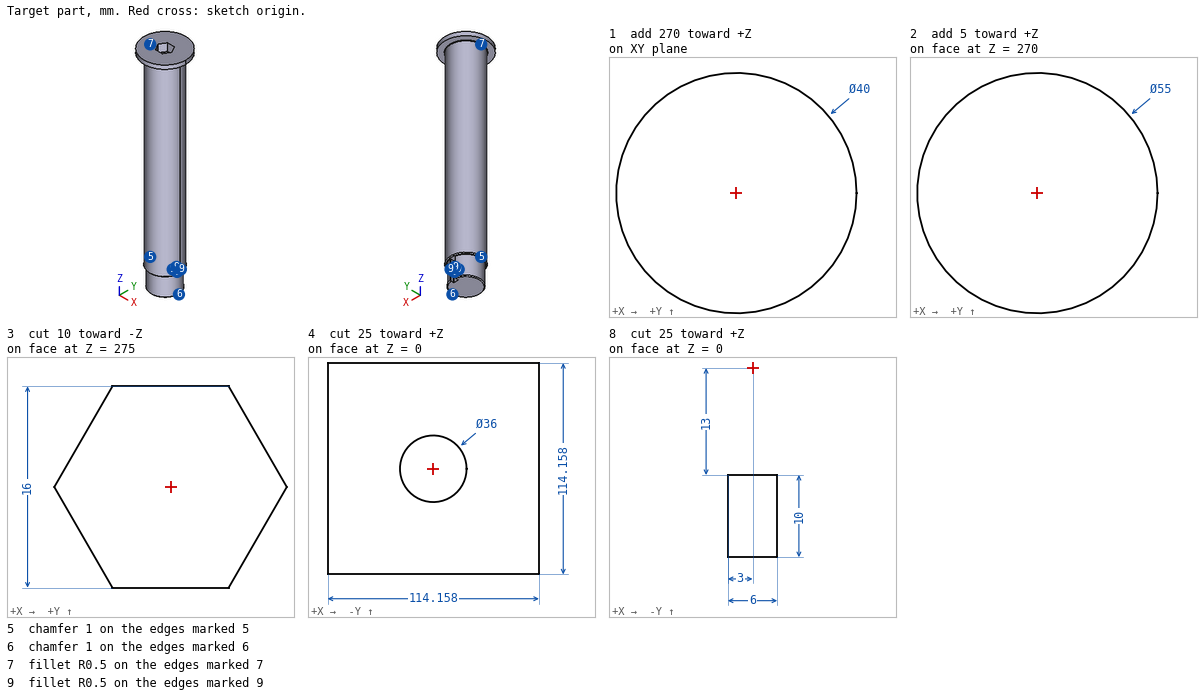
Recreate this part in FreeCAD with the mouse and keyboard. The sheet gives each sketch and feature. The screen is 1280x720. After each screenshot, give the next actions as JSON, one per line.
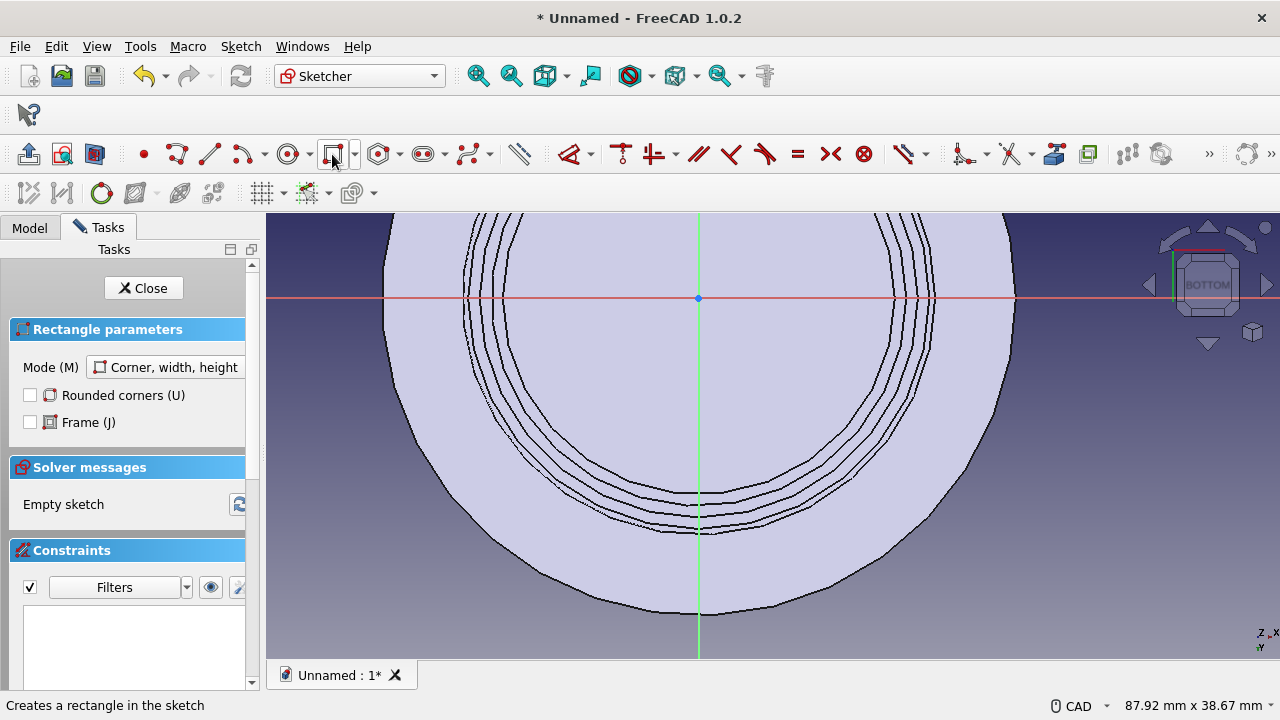
{"action": "left_click", "coordinate": [664, 448]}
{"action": "mouse_move", "coordinate": [733, 564]}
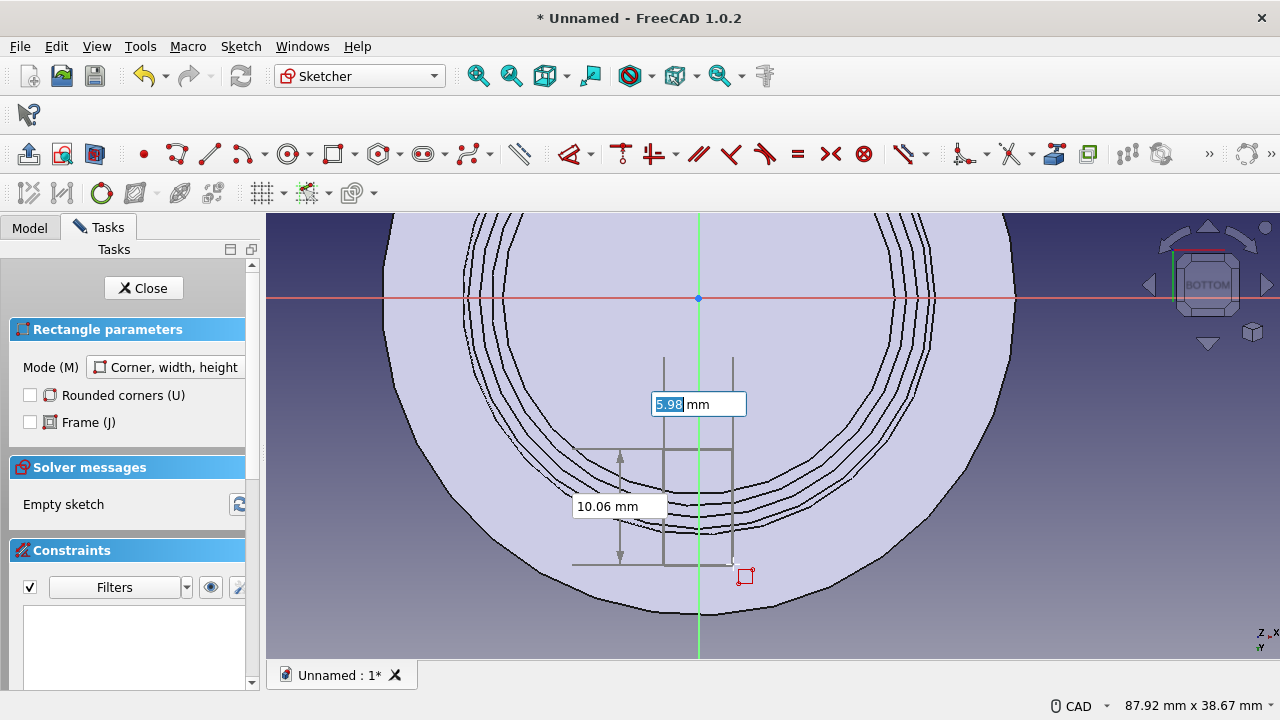
{"action": "type", "text": "6"}
{"action": "key", "text": "Tab"}
{"action": "type", "text": "10"}
{"action": "key", "text": "Return"}
{"action": "key", "text": "Escape"}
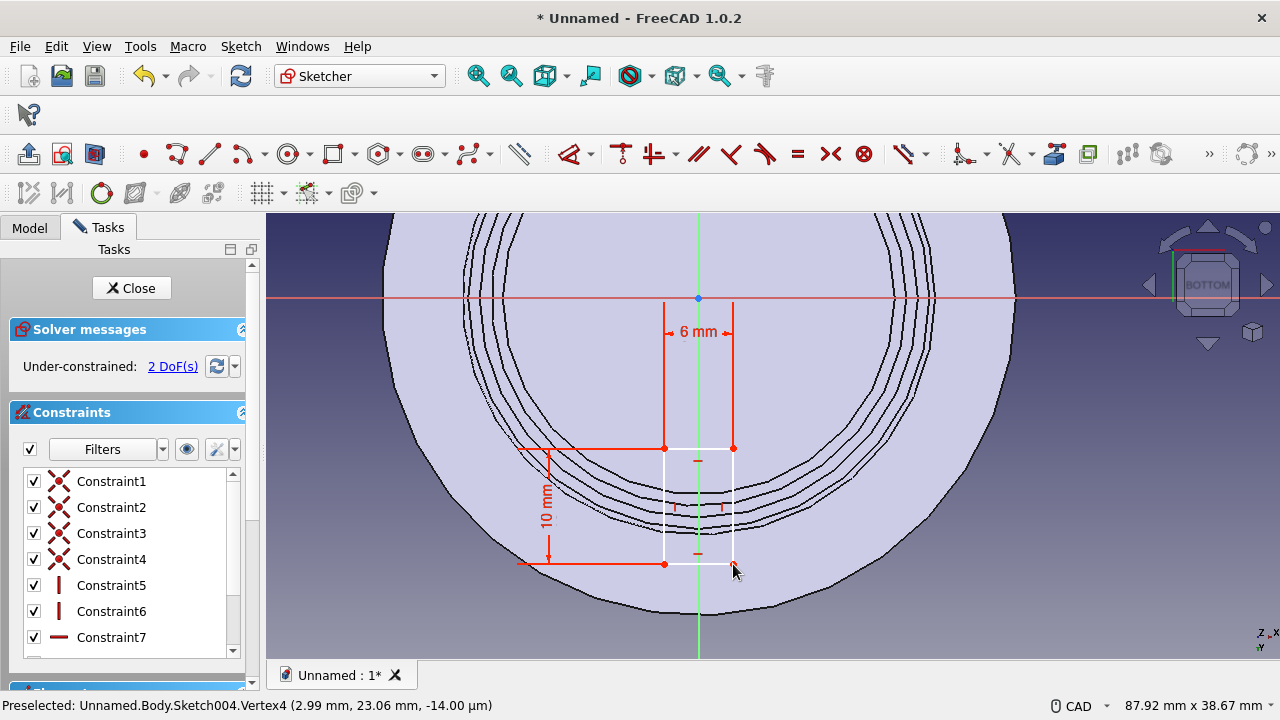
{"action": "left_click", "coordinate": [568, 154]}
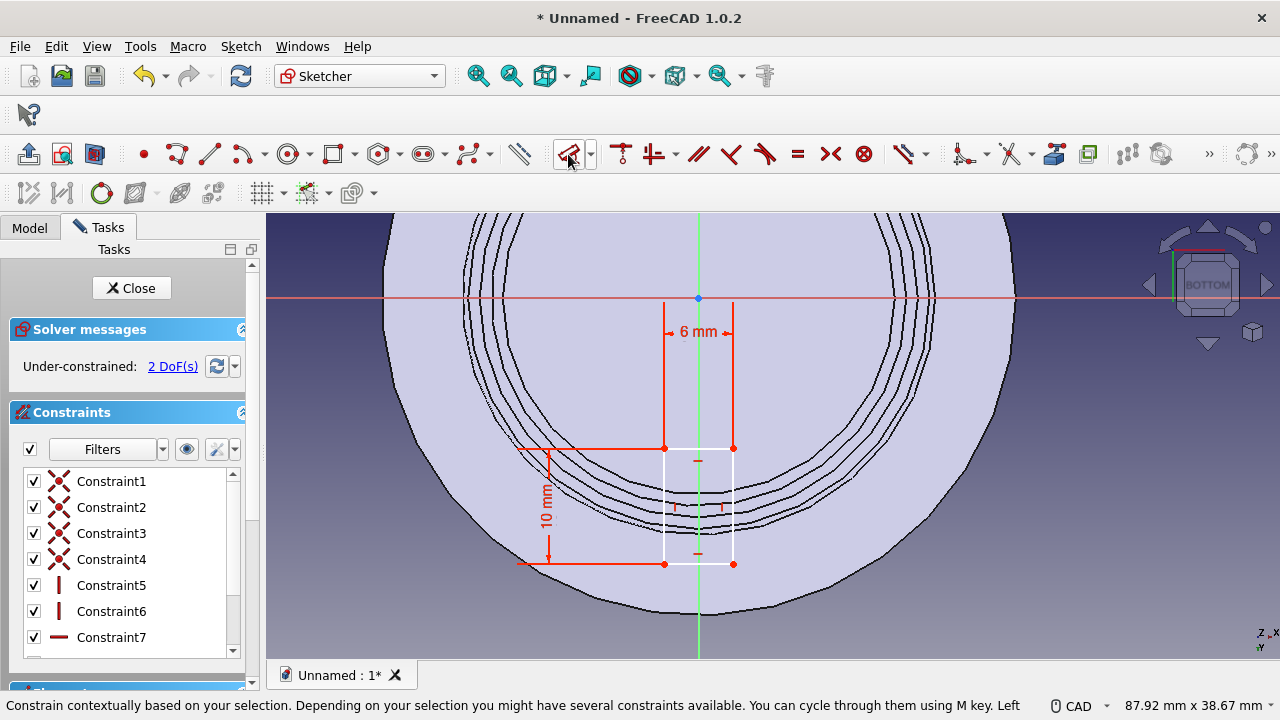
{"action": "left_click", "coordinate": [664, 449]}
{"action": "left_click", "coordinate": [681, 264]}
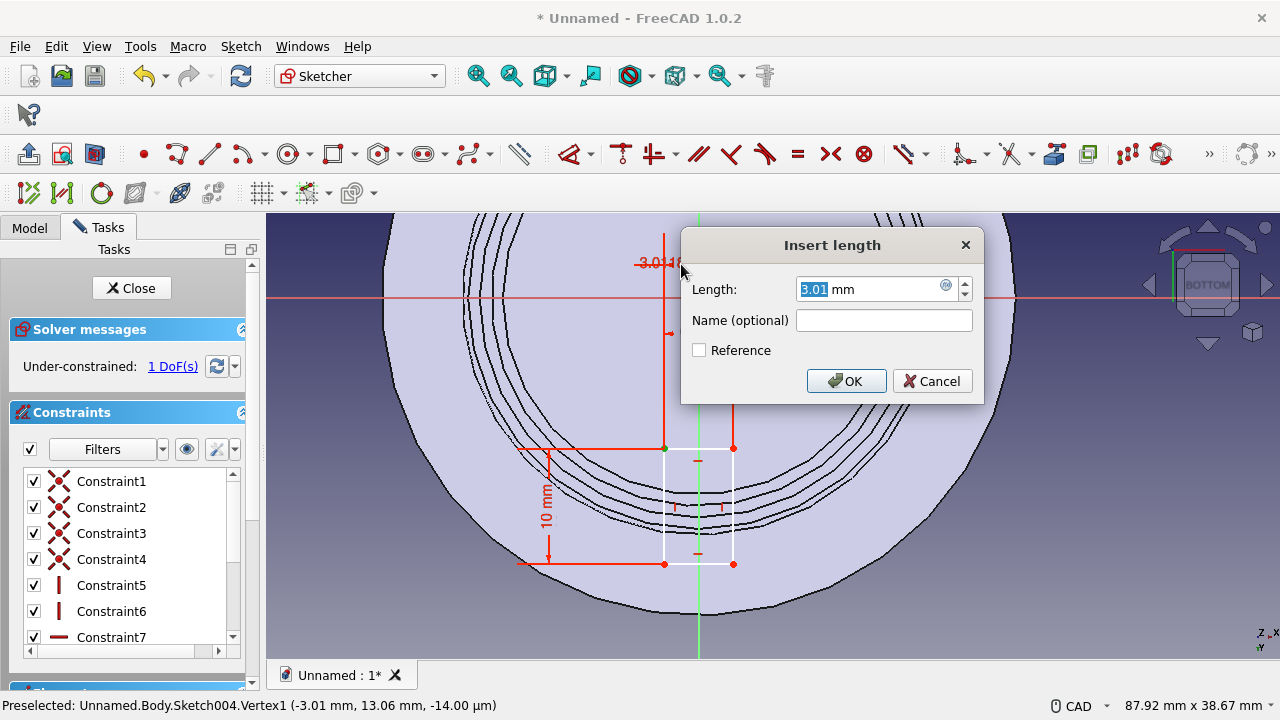
{"action": "type", "text": "3"}
{"action": "key", "text": "Return"}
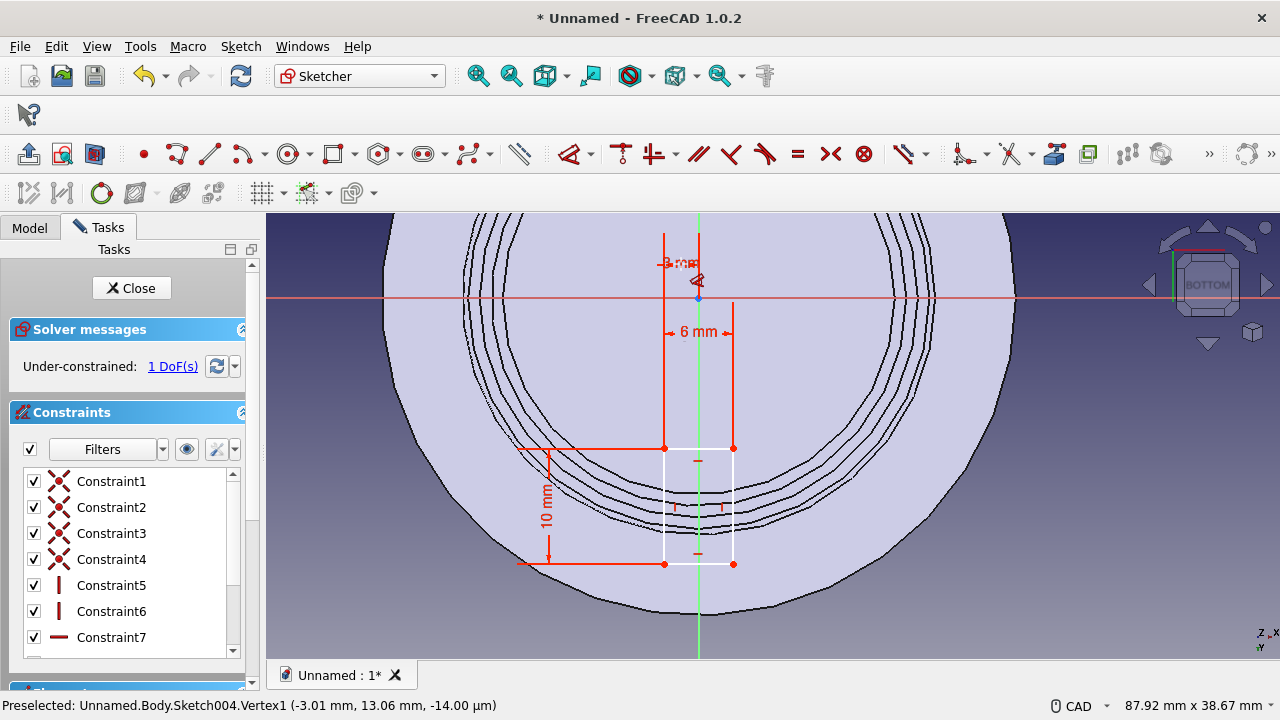
{"action": "left_click", "coordinate": [664, 449]}
{"action": "left_click", "coordinate": [630, 374]}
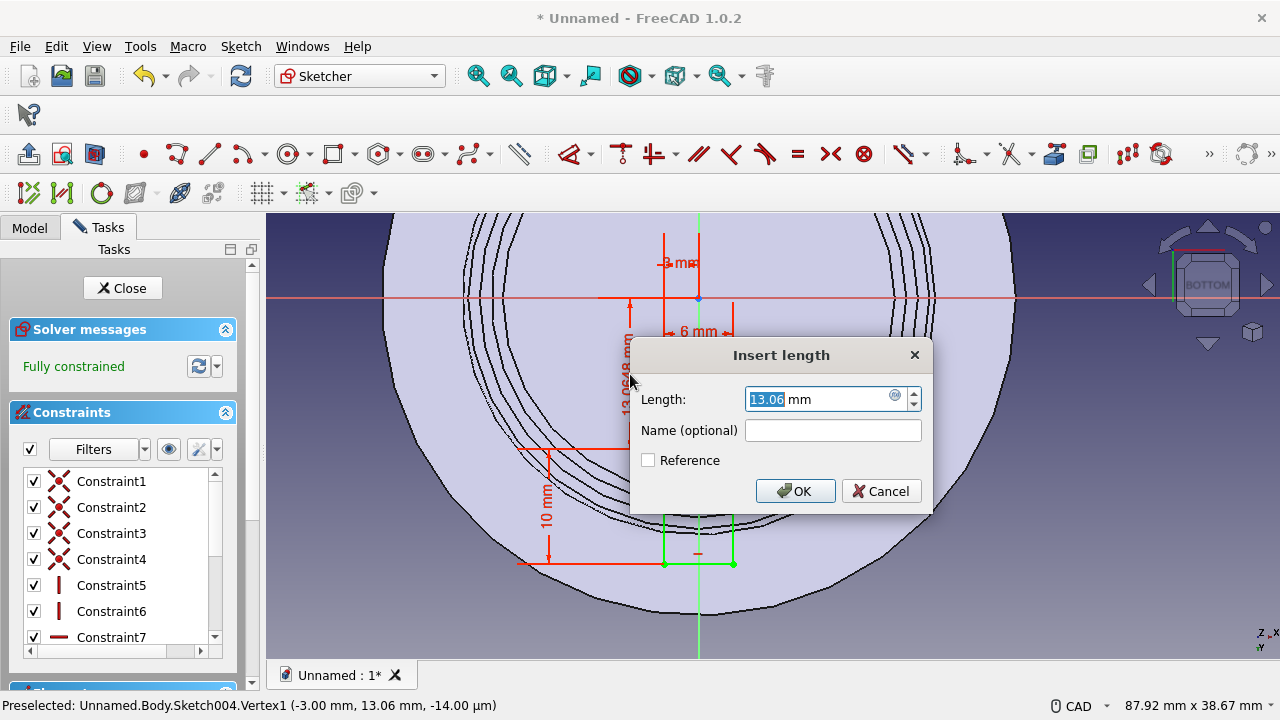
{"action": "type", "text": "13"}
{"action": "key", "text": "Return"}
{"action": "key", "text": "Escape"}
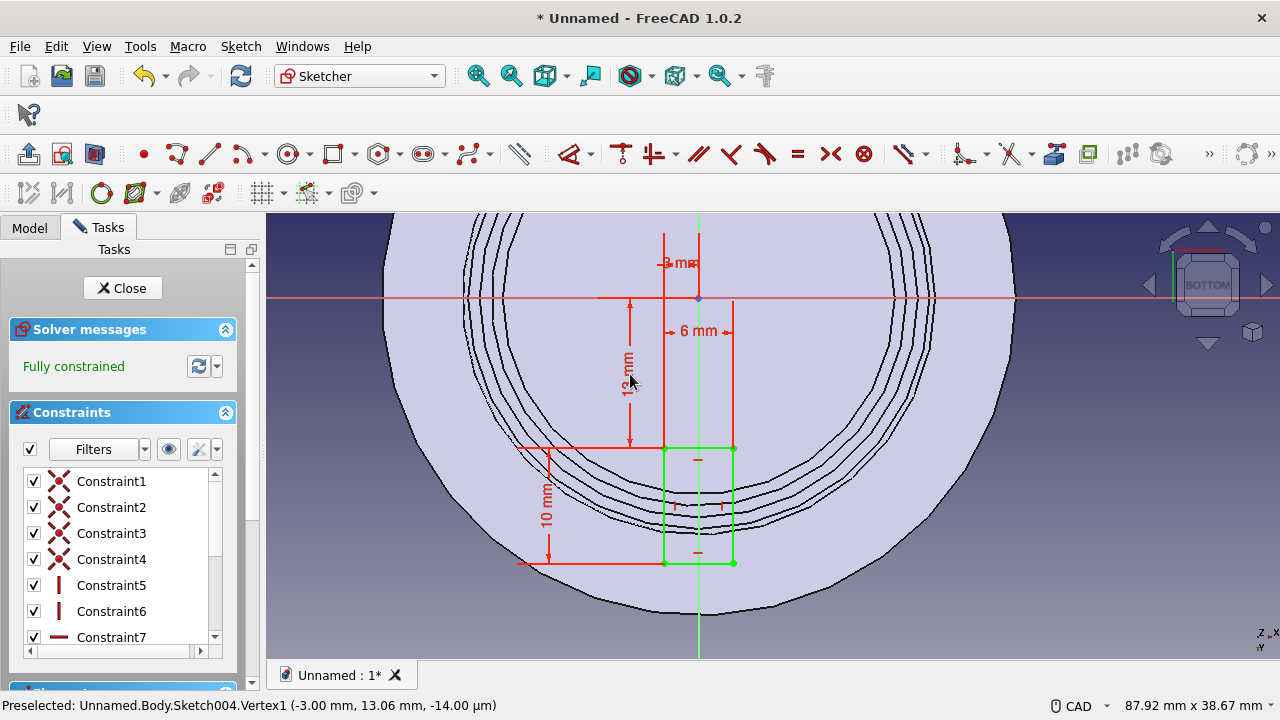
{"action": "left_click", "coordinate": [123, 288]}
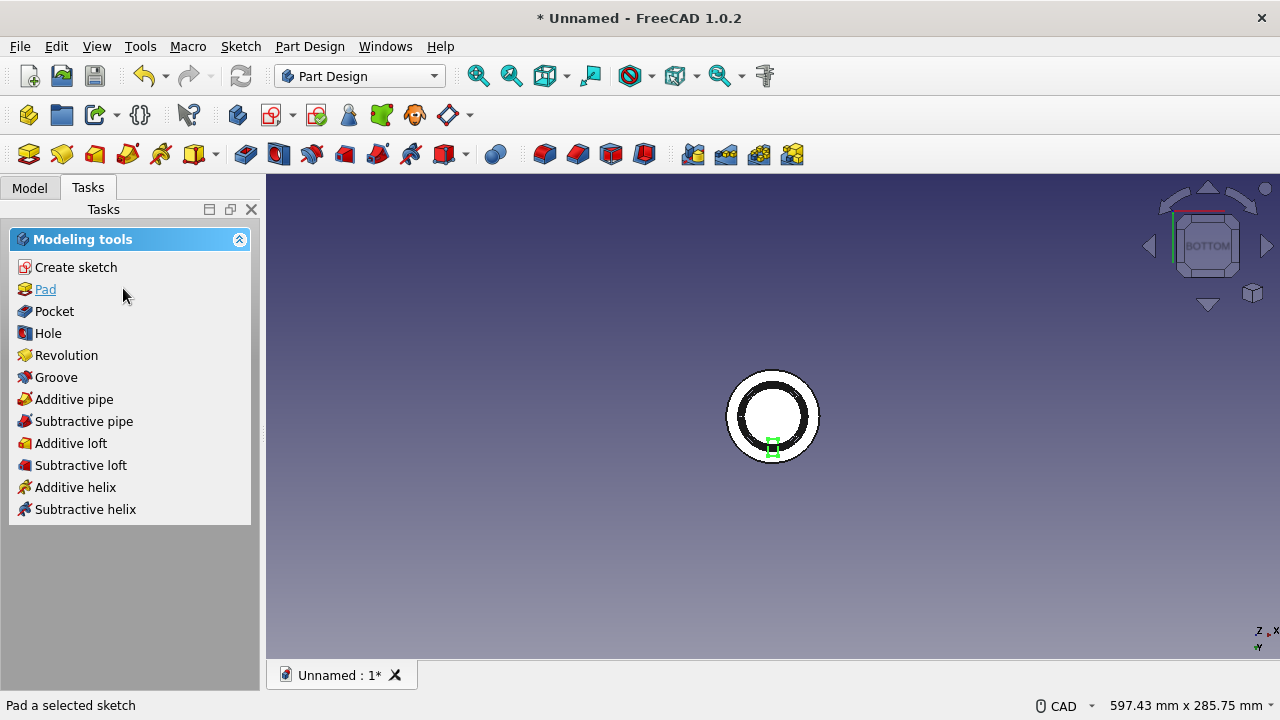
{"action": "left_click", "coordinate": [246, 154]}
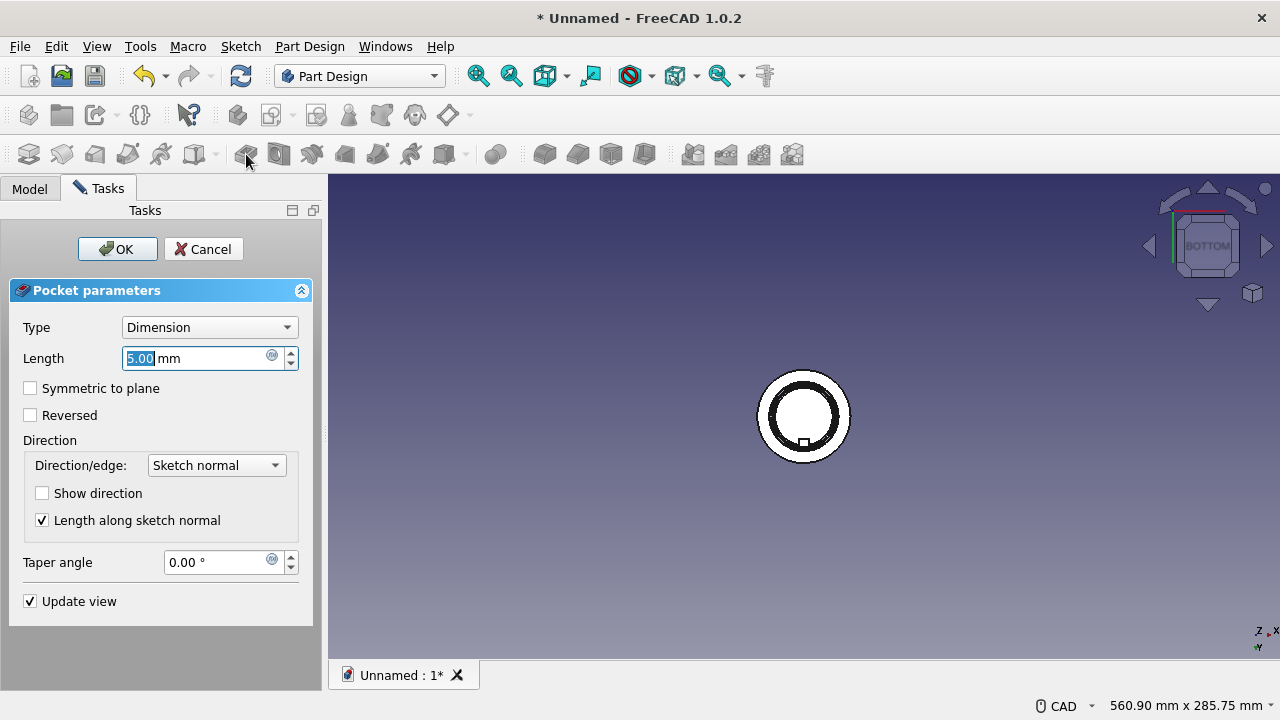
{"action": "type", "text": "25"}
{"action": "key", "text": "Tab"}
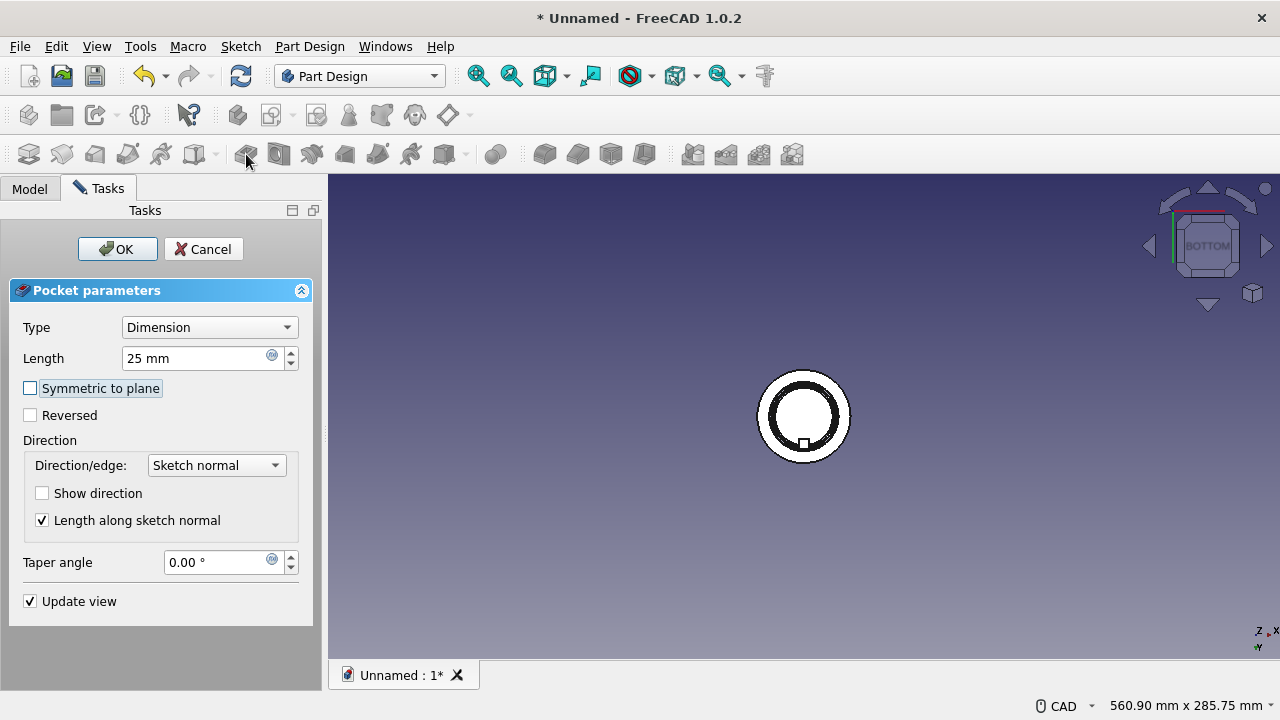
{"action": "left_click", "coordinate": [118, 249]}